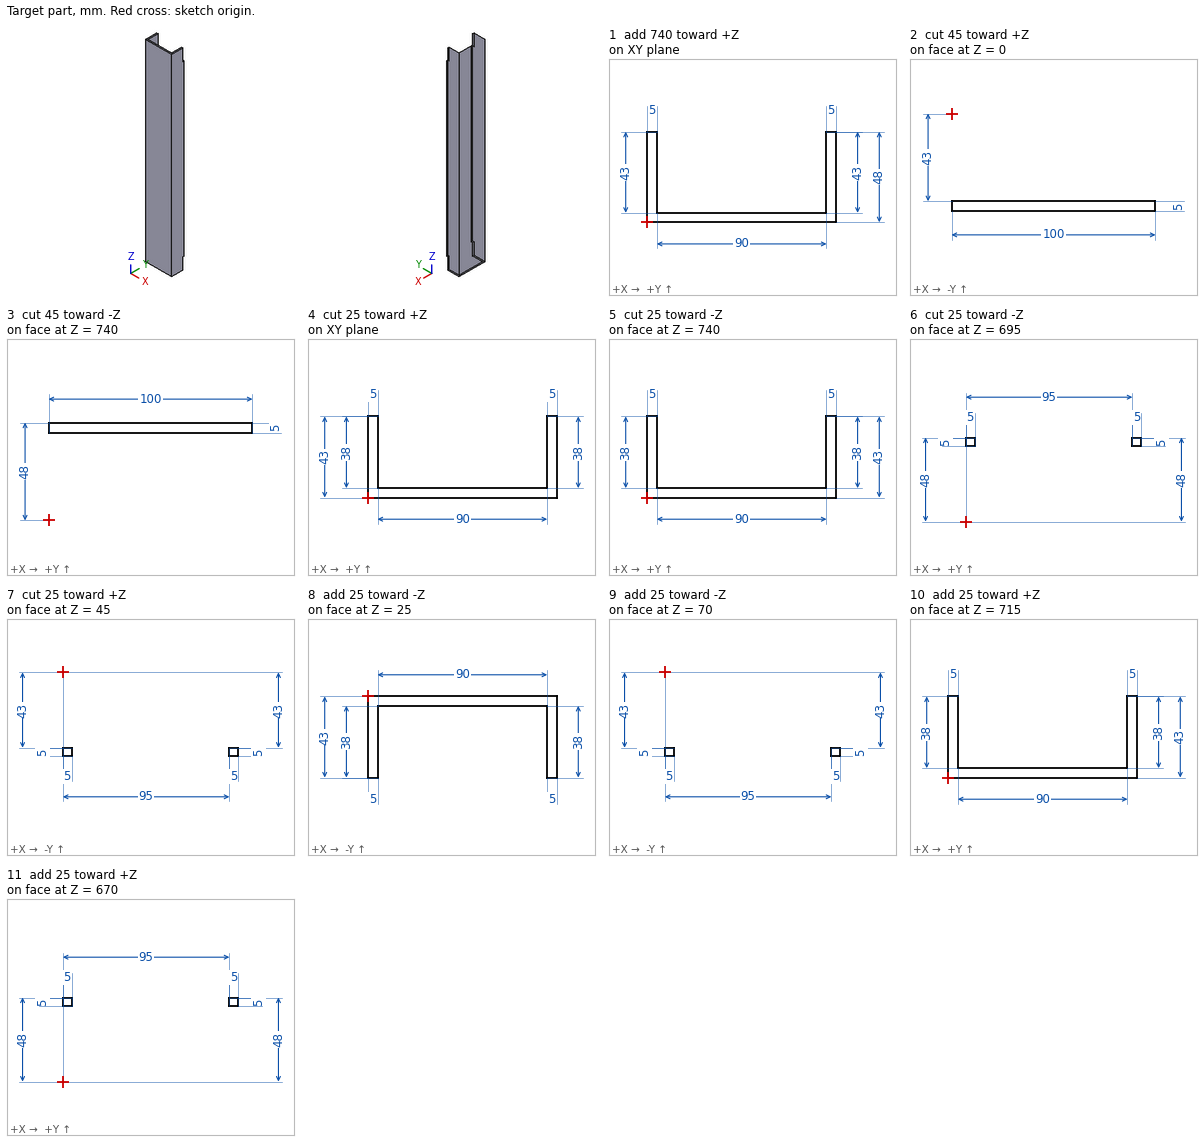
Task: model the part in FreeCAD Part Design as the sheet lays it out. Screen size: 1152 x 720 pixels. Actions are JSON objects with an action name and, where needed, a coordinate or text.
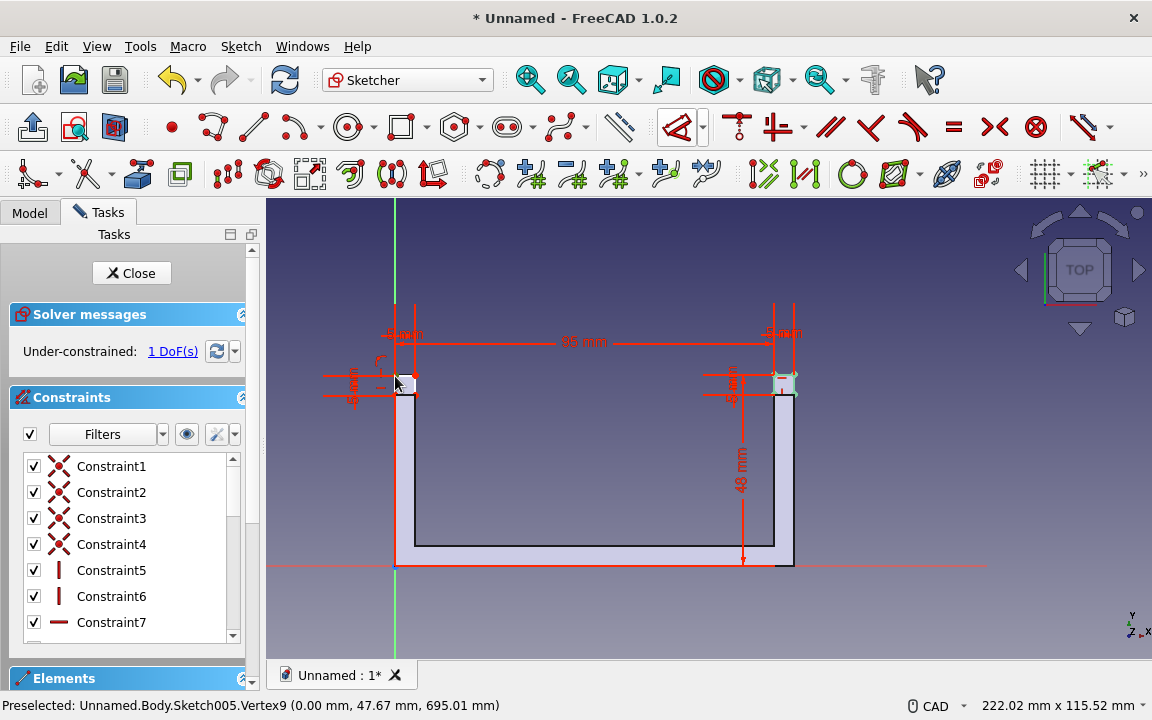
{"action": "key", "text": "i"}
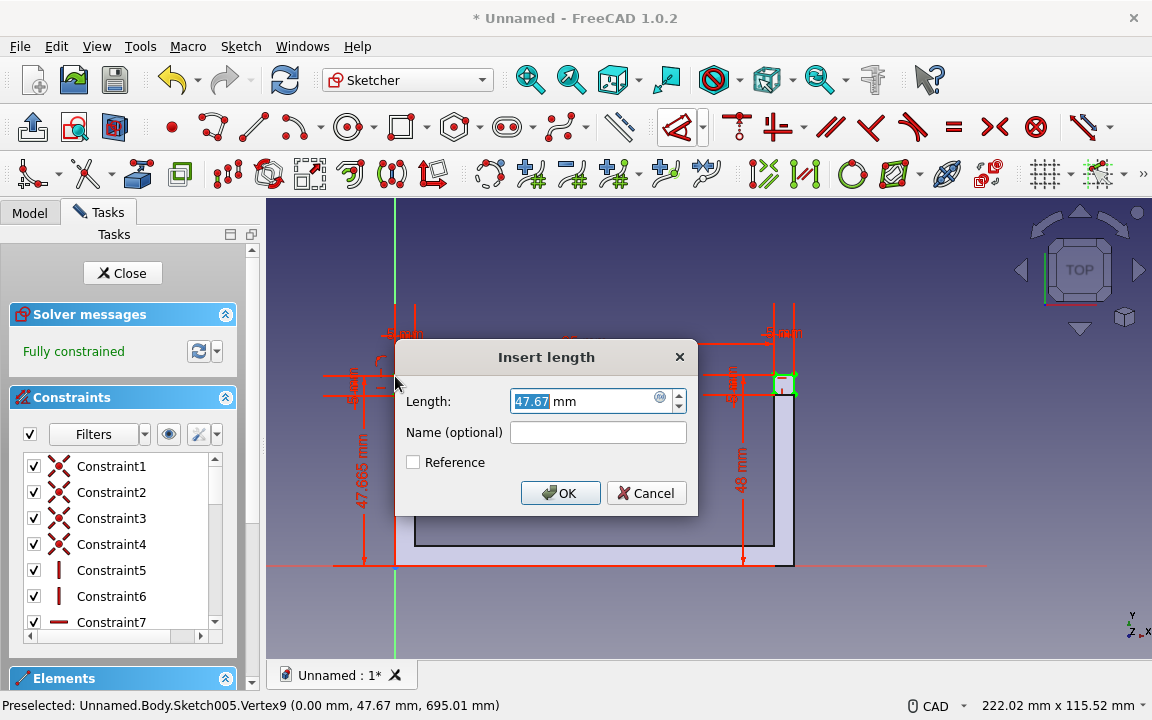
{"action": "type", "text": "48"}
{"action": "key", "text": "Return"}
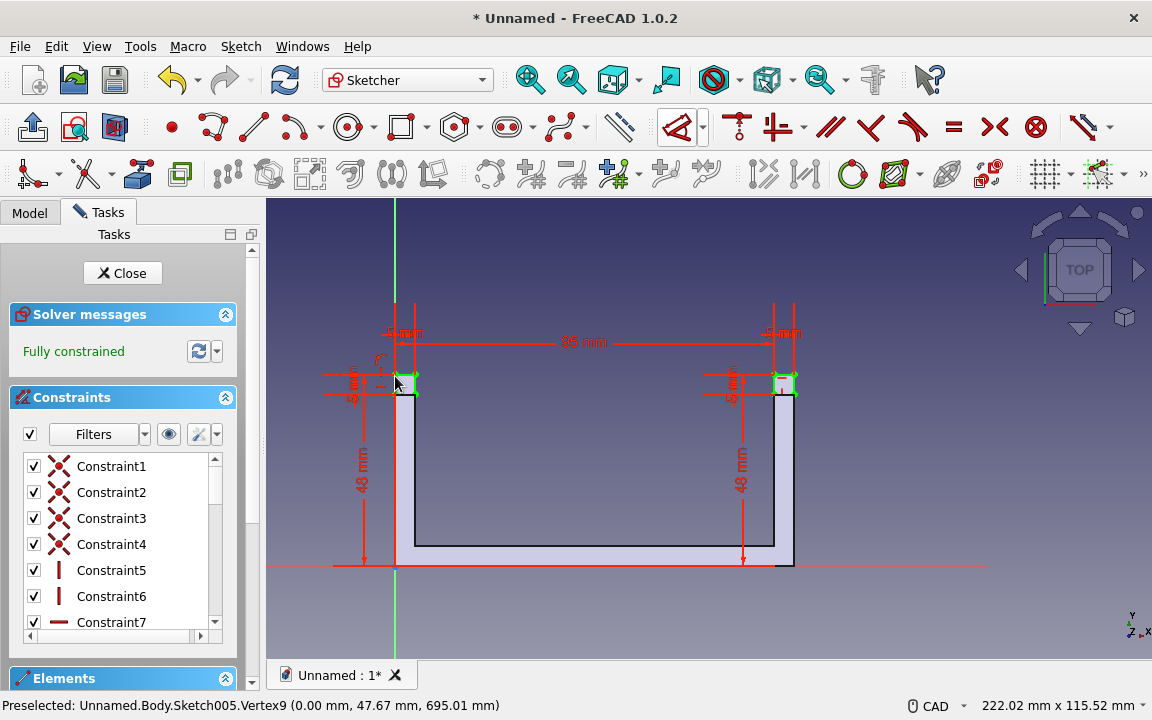
{"action": "left_click", "coordinate": [123, 273]}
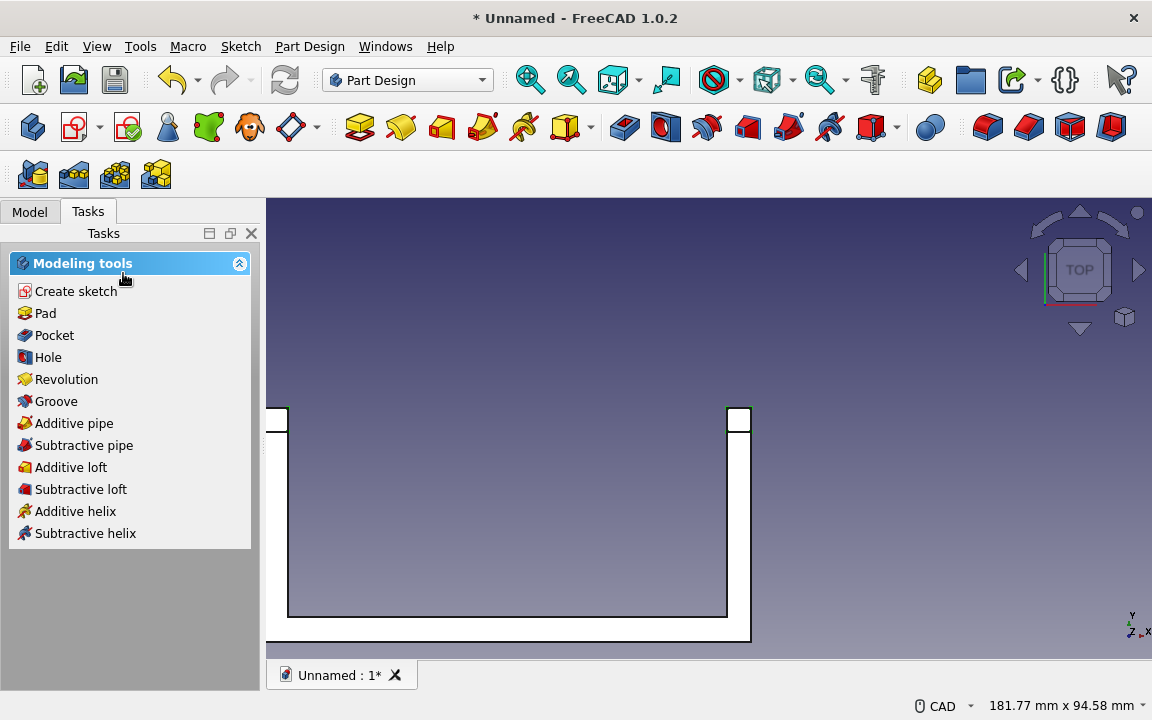
{"action": "left_click", "coordinate": [625, 128]}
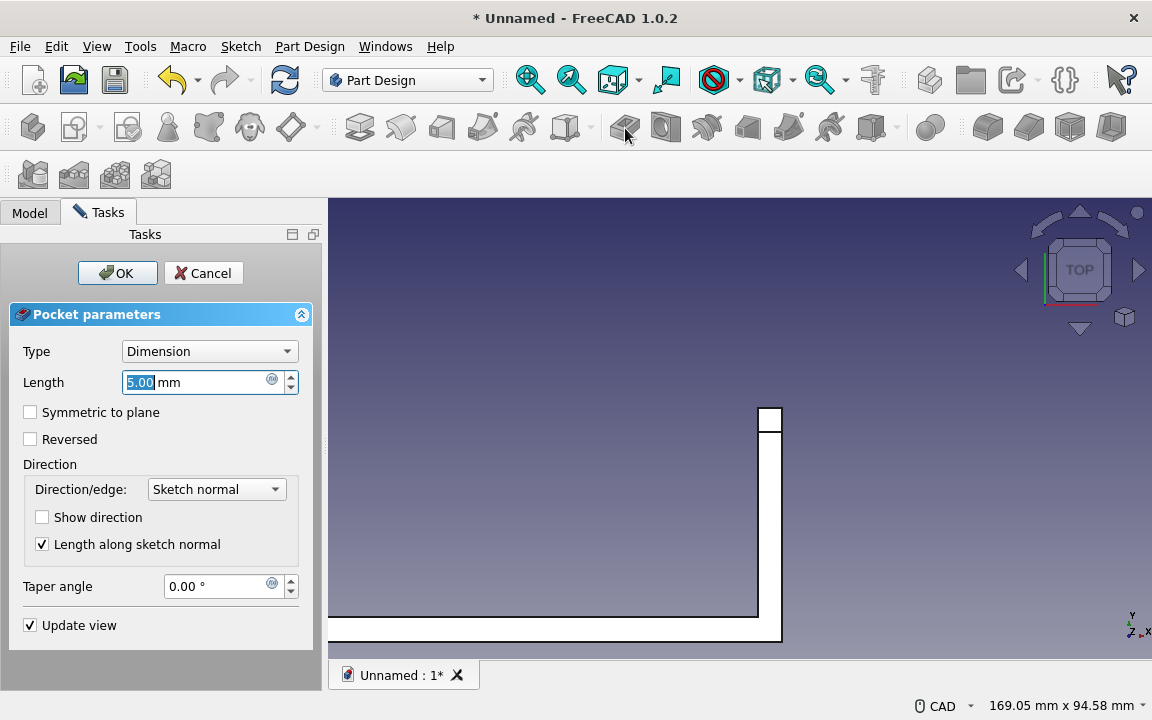
{"action": "type", "text": "25"}
{"action": "key", "text": "Tab"}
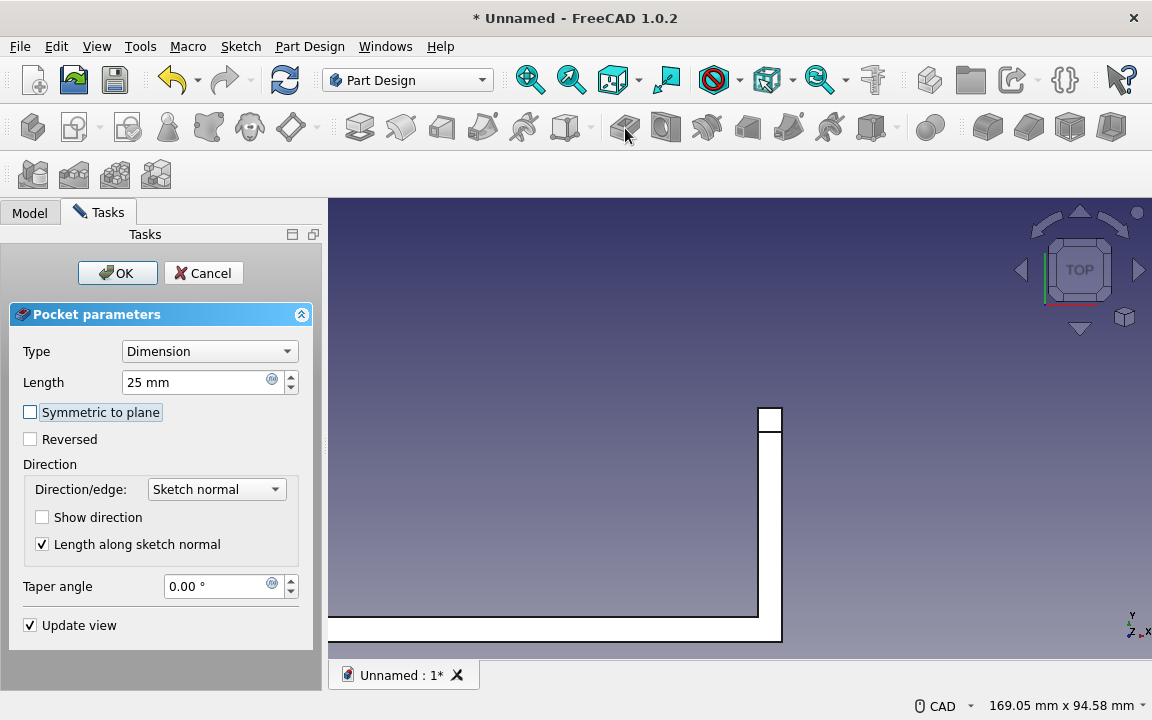
{"action": "left_click", "coordinate": [118, 273]}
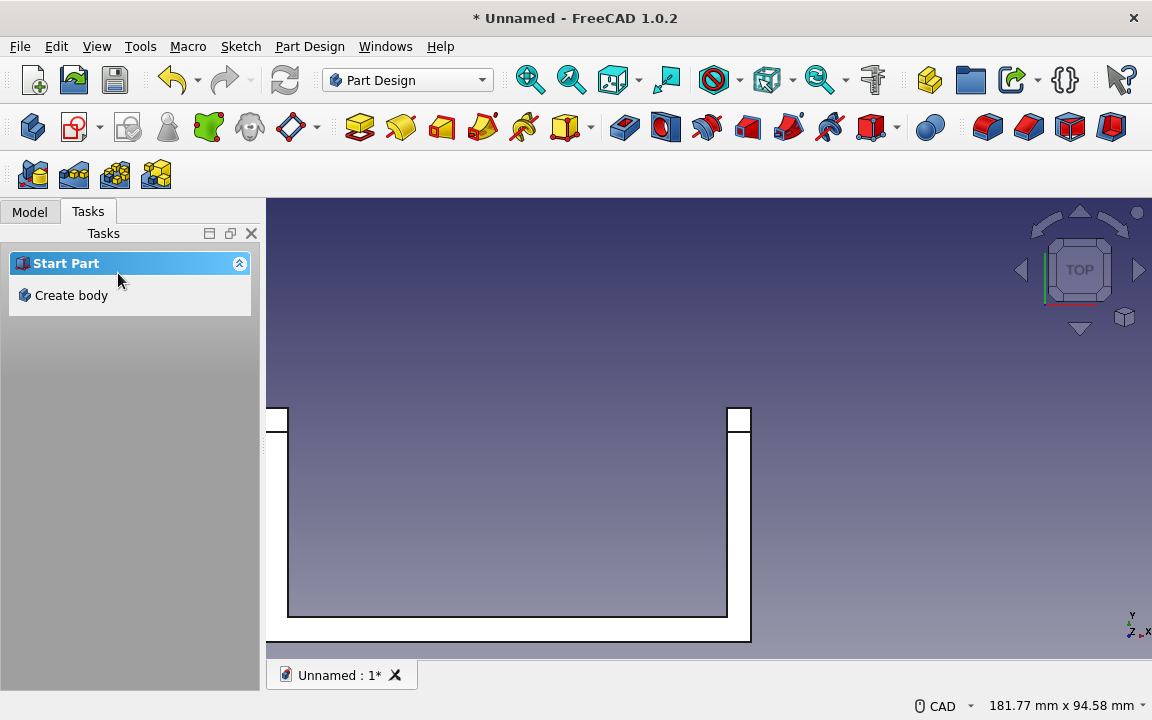
{"action": "left_click", "coordinate": [531, 80]}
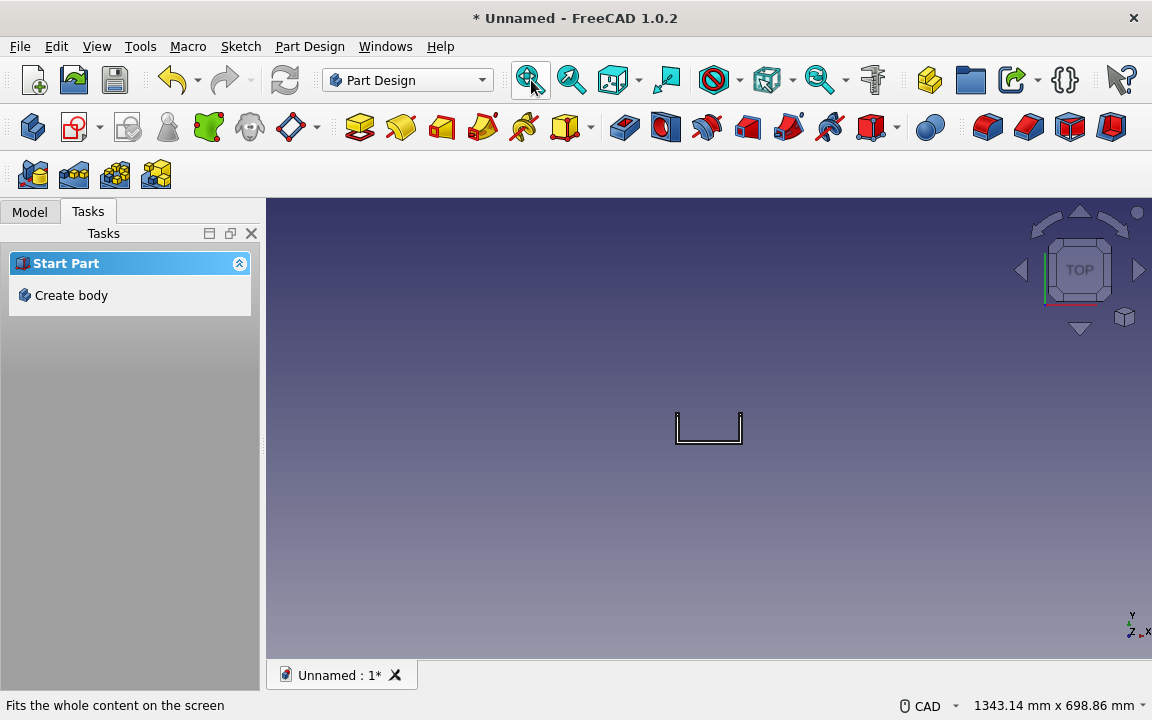
{"action": "key", "text": "5"}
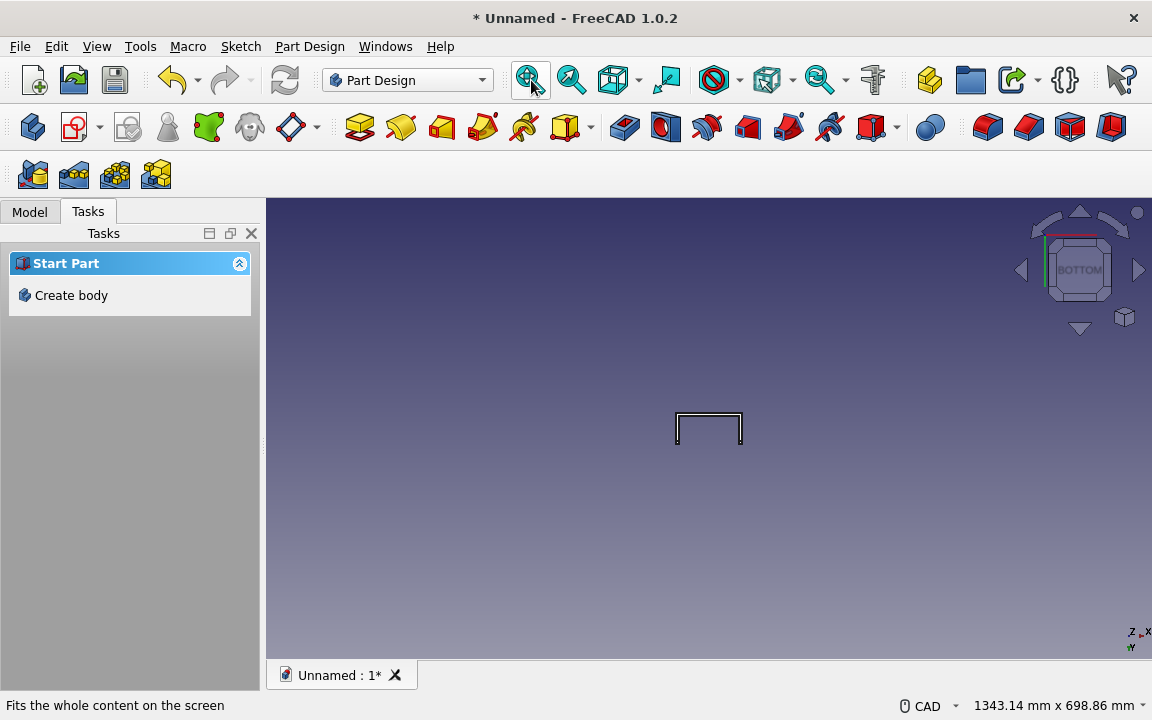
{"action": "left_click", "coordinate": [531, 80]}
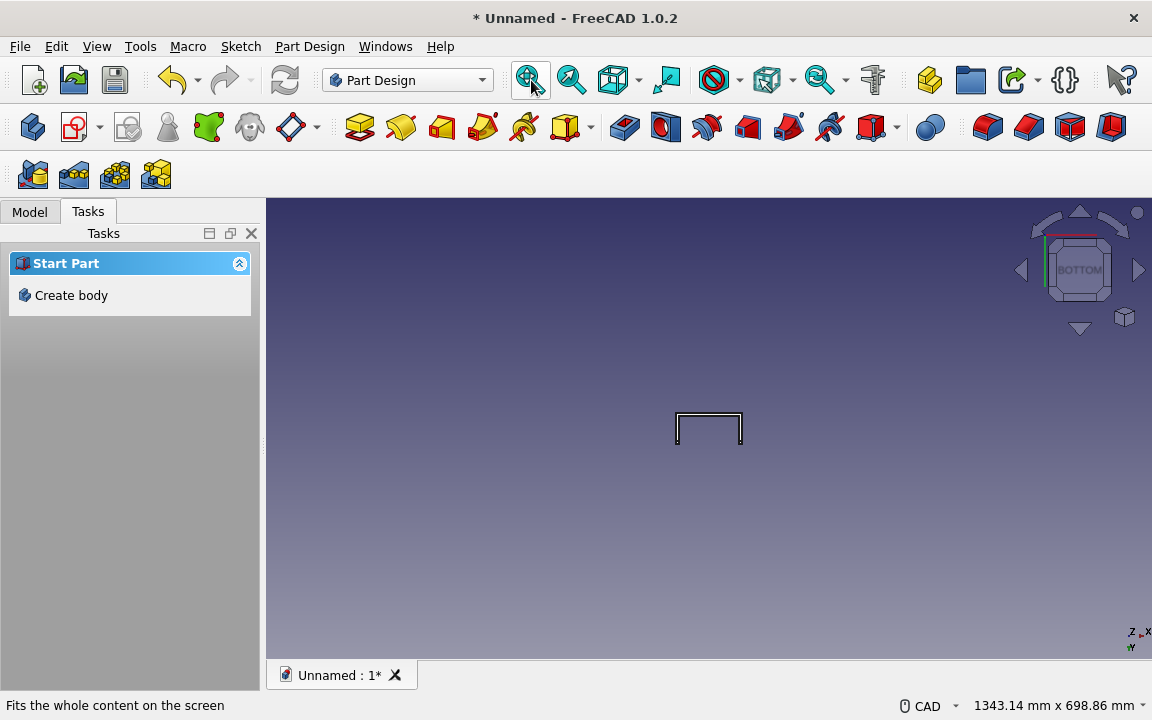
{"action": "scroll", "coordinate": [740, 442], "scroll_direction": "up", "scroll_amount": 10}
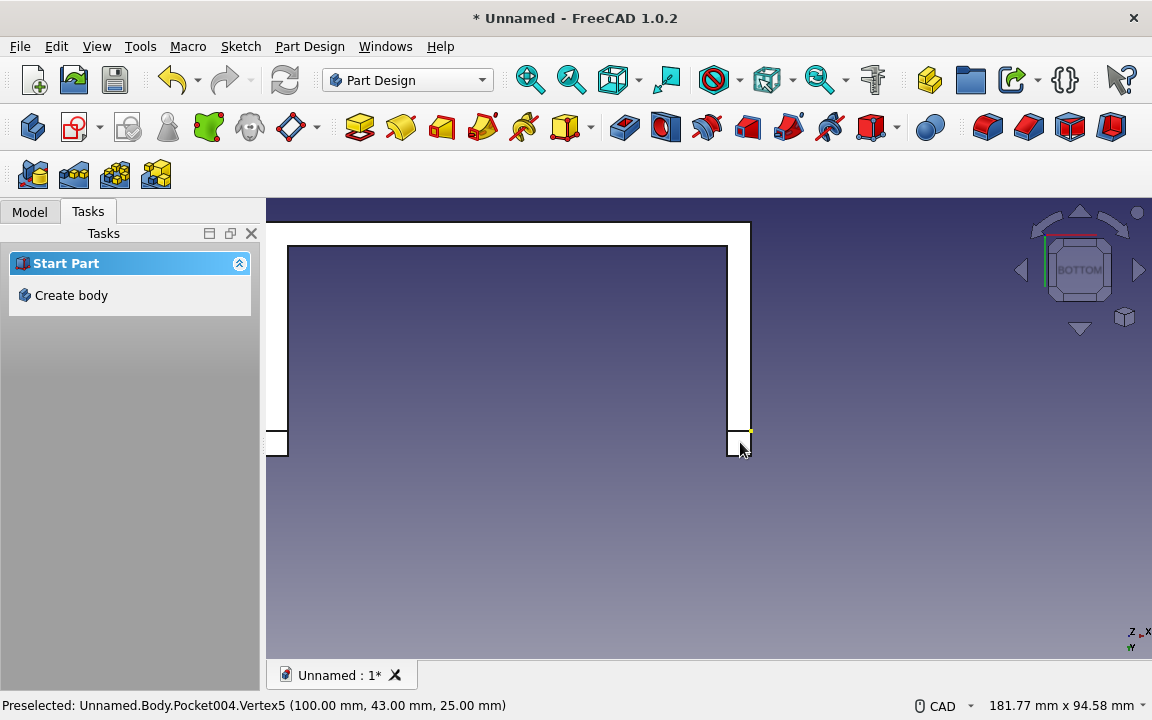
{"action": "left_click", "coordinate": [739, 443]}